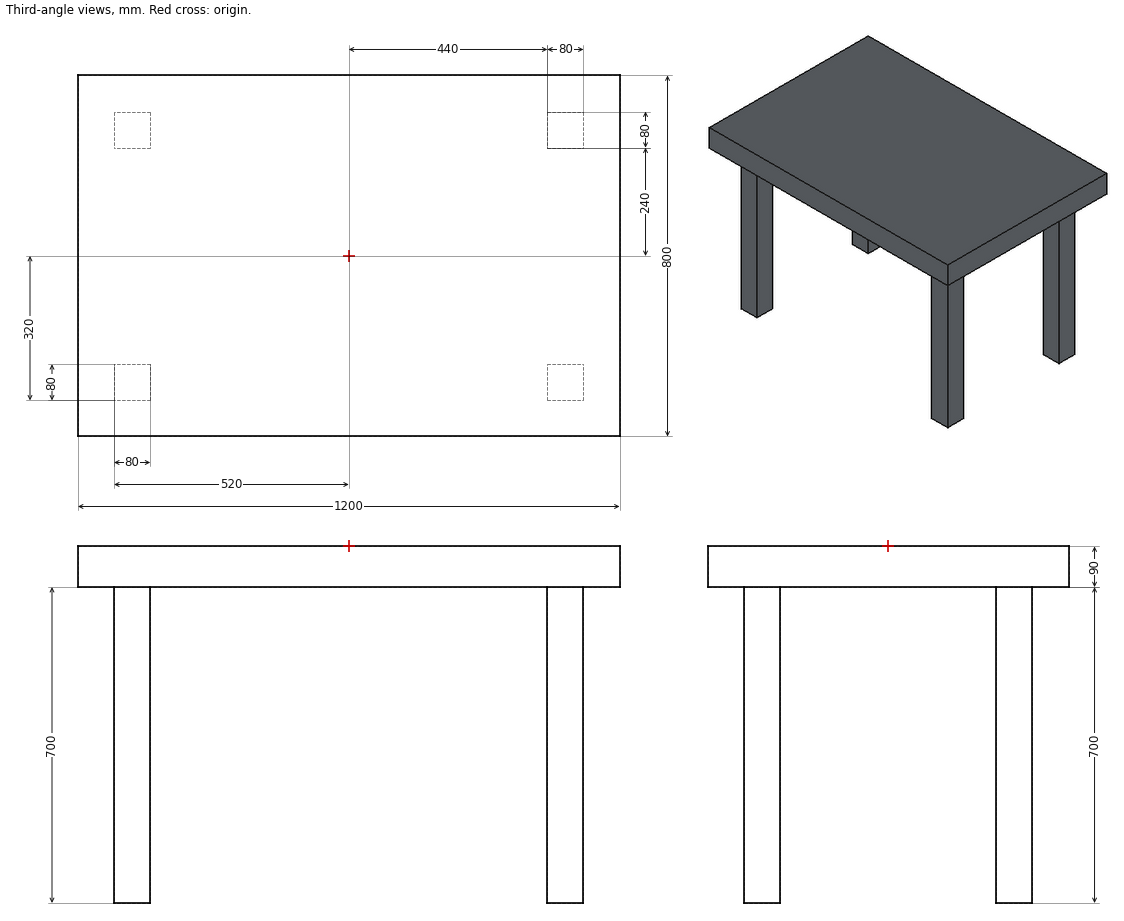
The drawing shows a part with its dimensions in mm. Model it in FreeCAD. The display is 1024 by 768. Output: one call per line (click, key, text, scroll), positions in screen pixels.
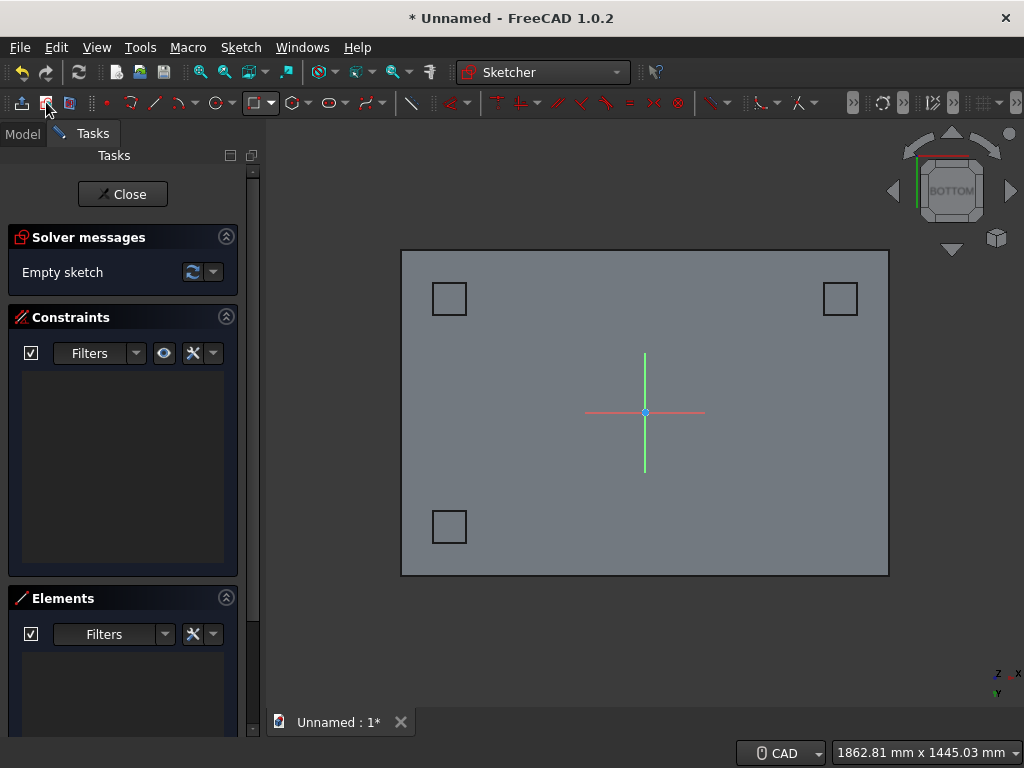
scroll(859, 538, up, 12)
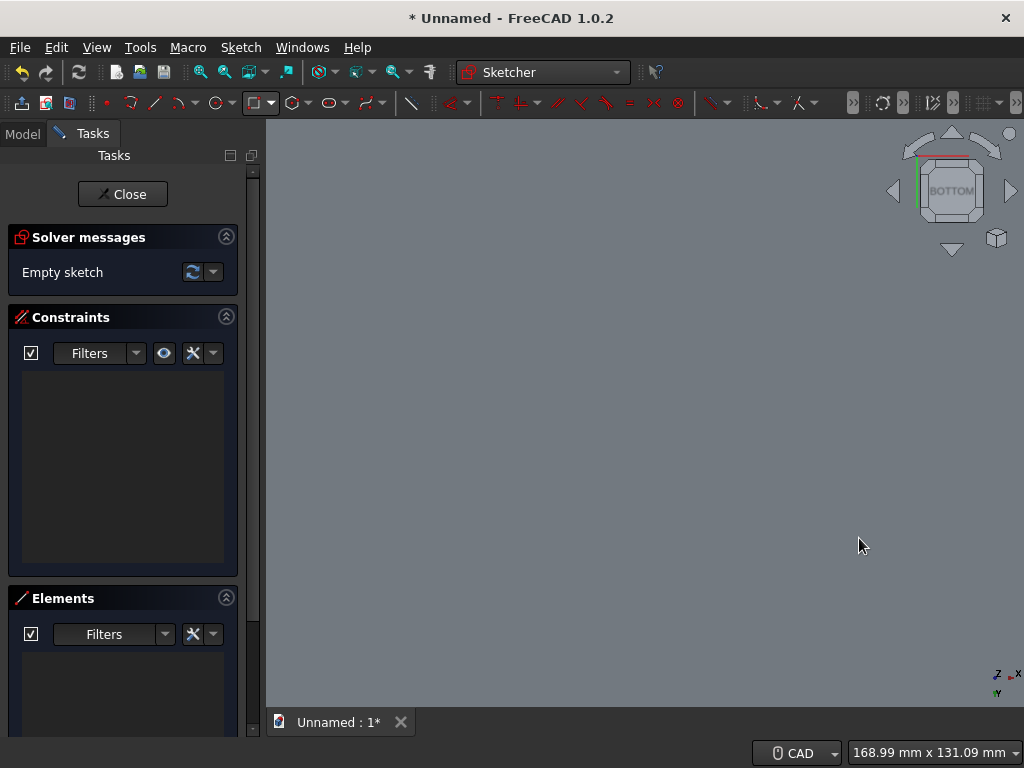
key(g)
key(r)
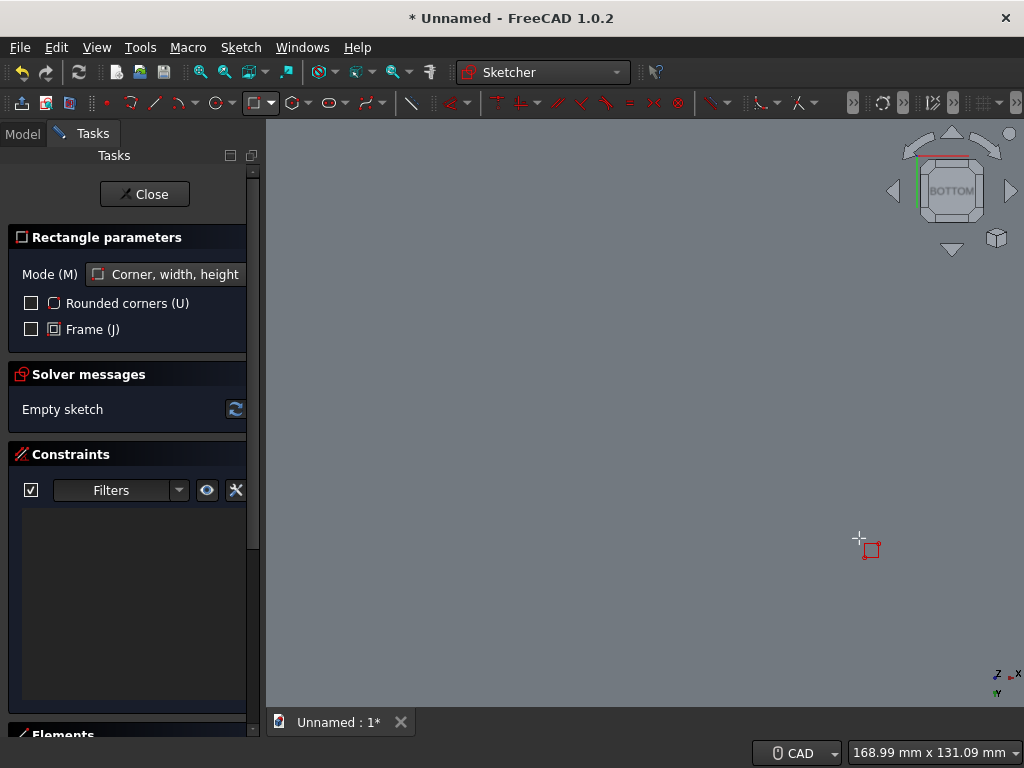
click(466, 229)
click(825, 588)
key(Escape)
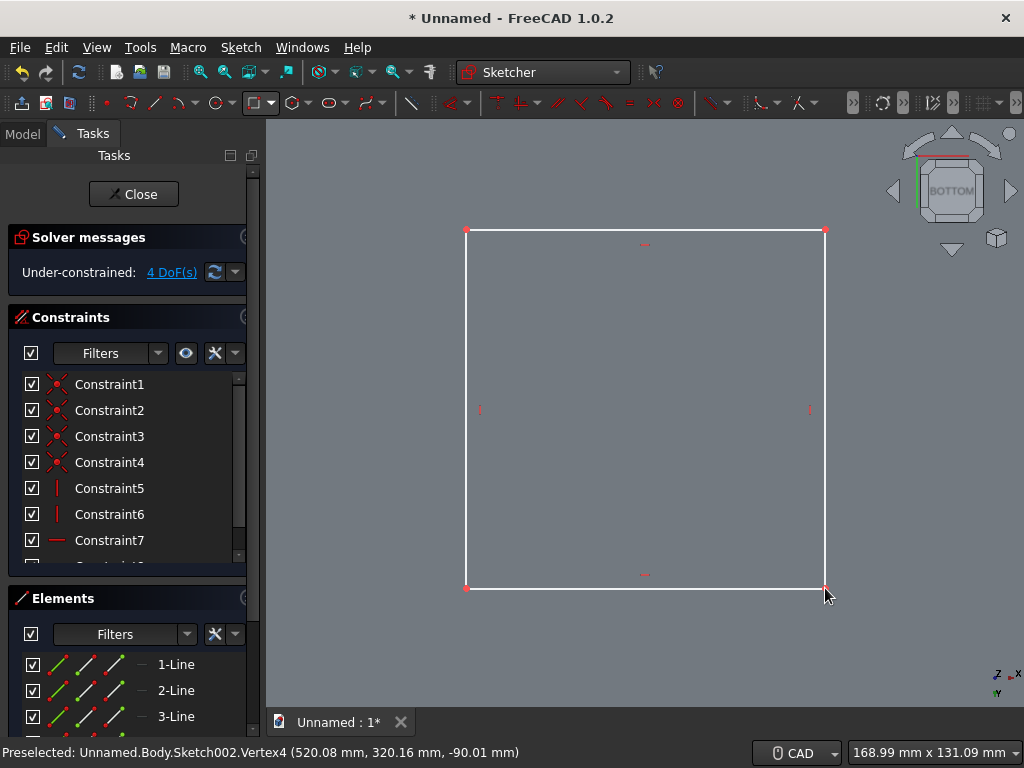
key(d)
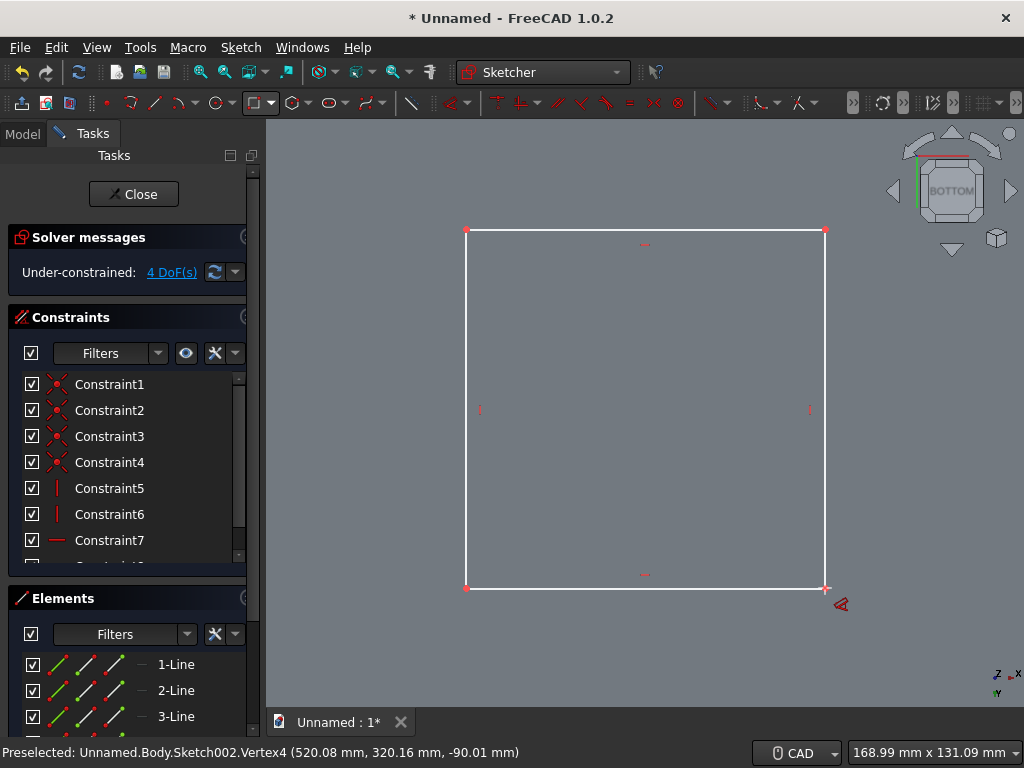
click(466, 338)
click(432, 410)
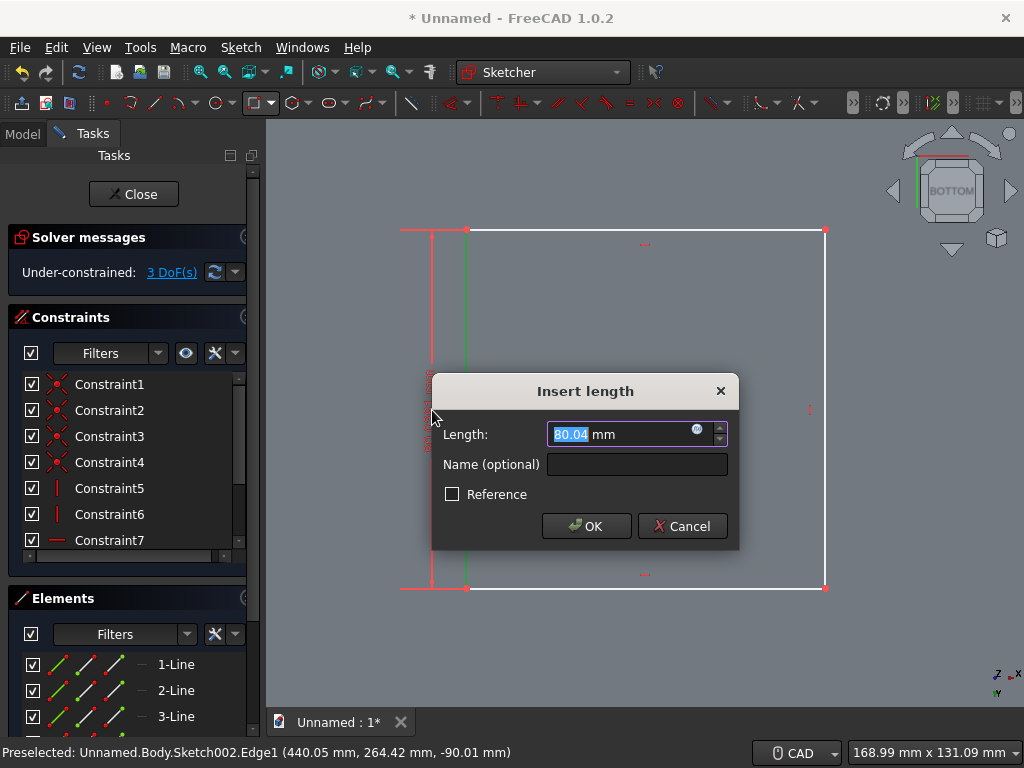
text(80)
key(Return)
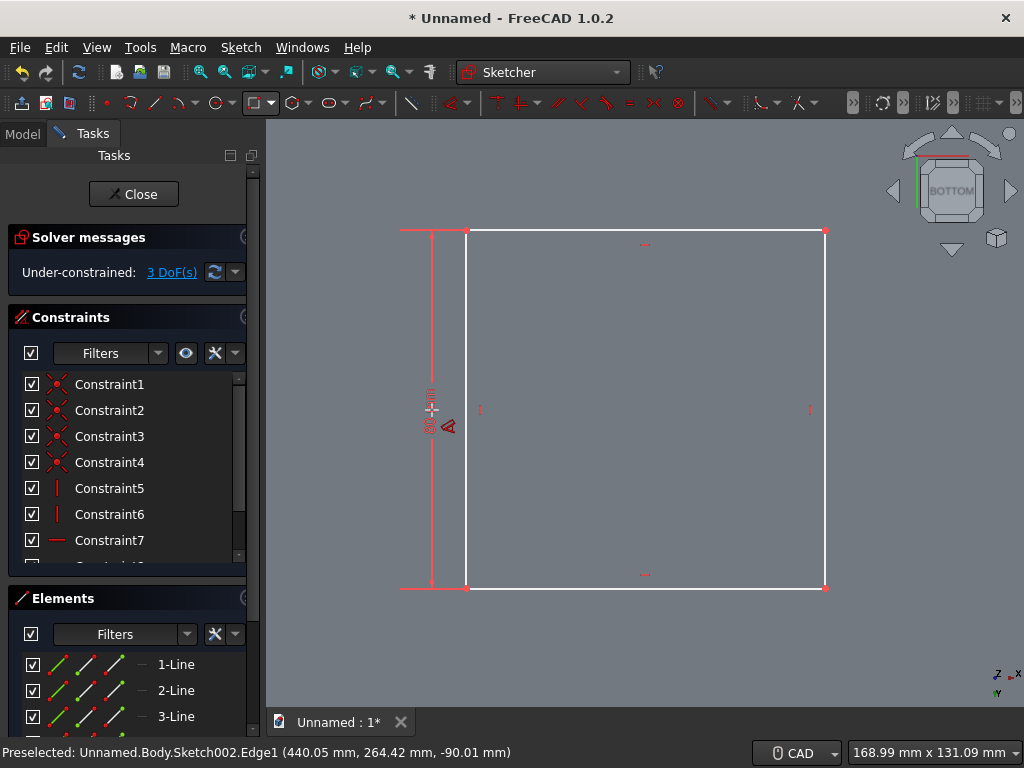
click(574, 589)
click(645, 623)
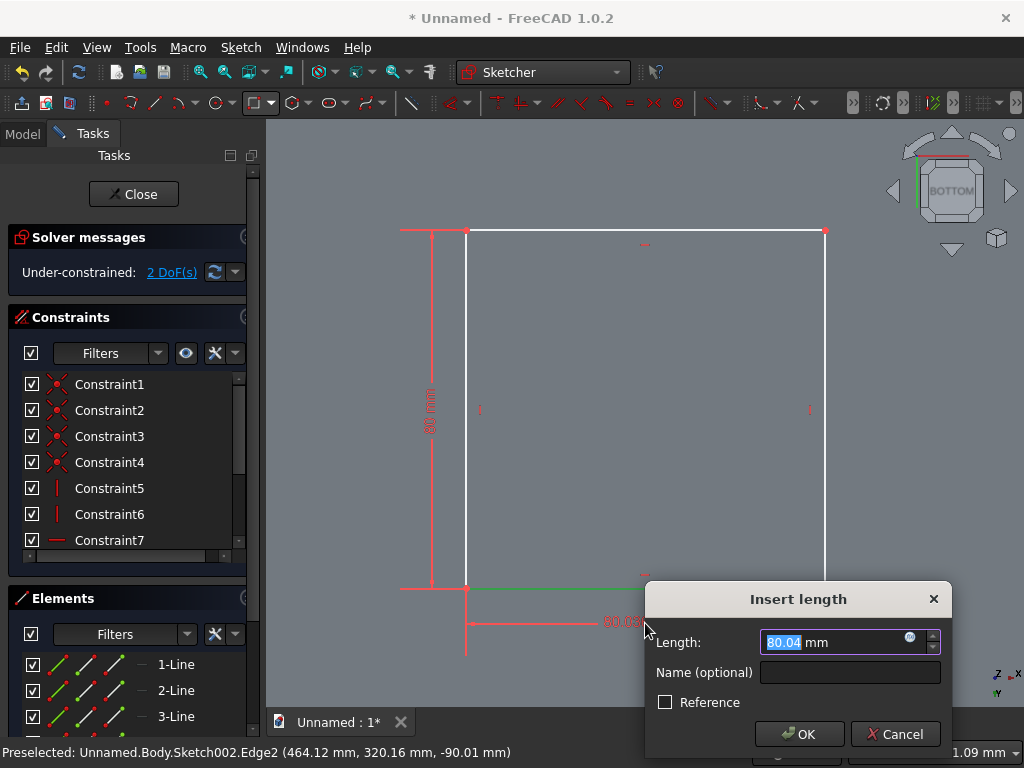
text(80)
key(Return)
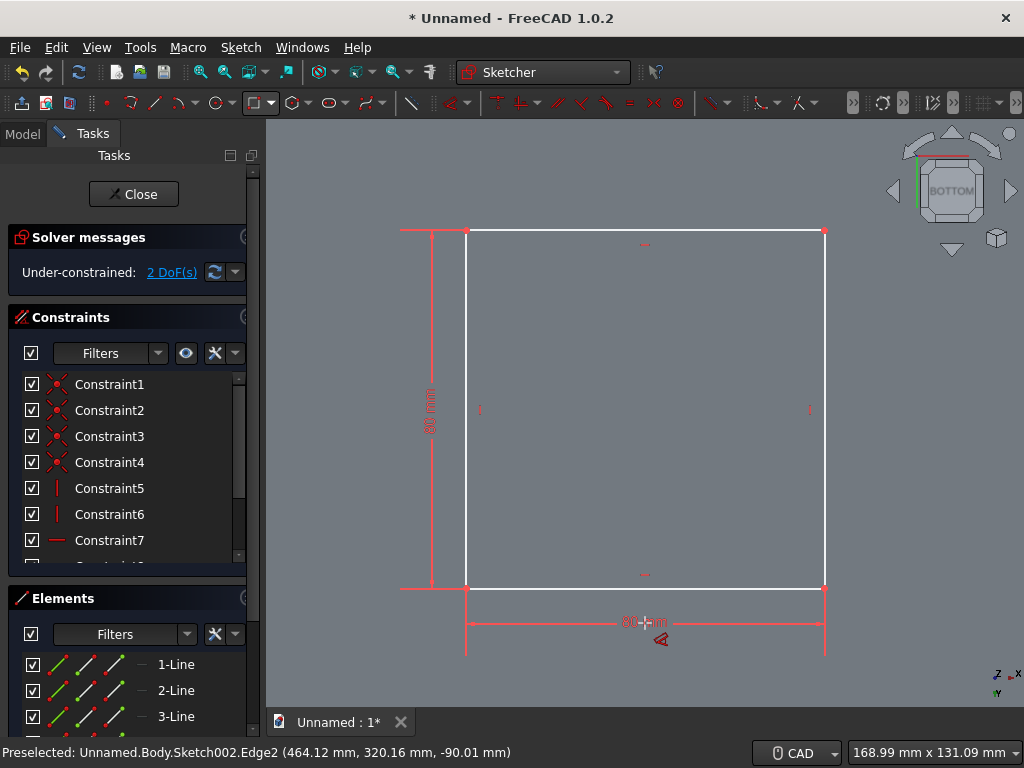
click(466, 230)
click(380, 264)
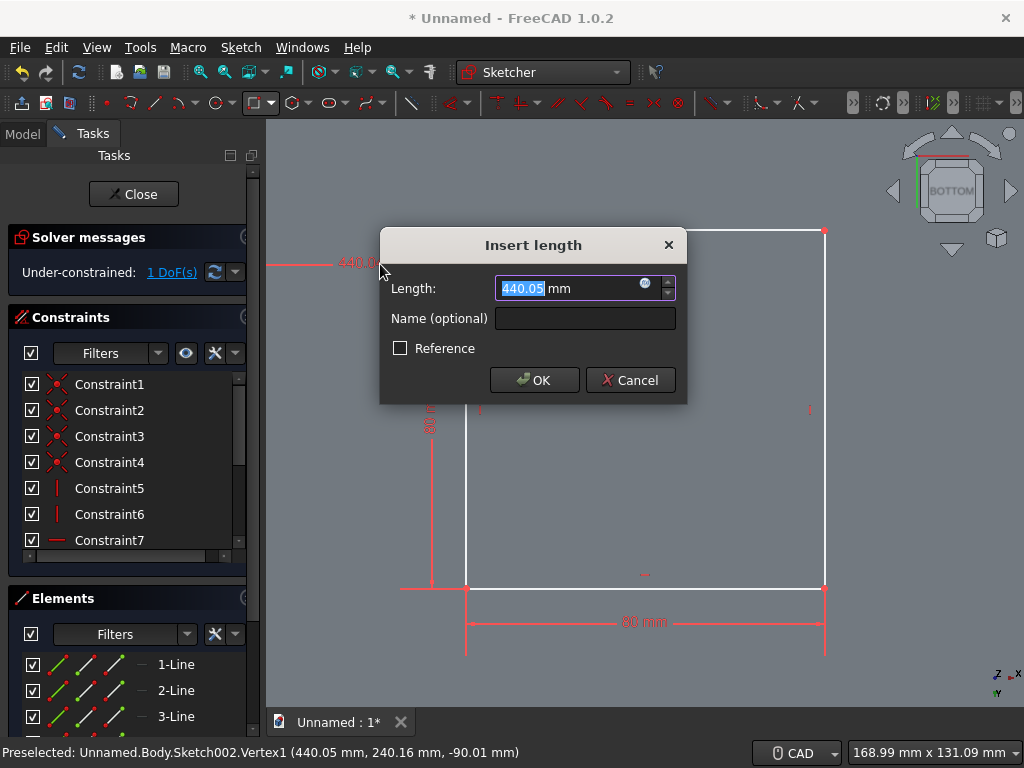
text(440)
key(Return)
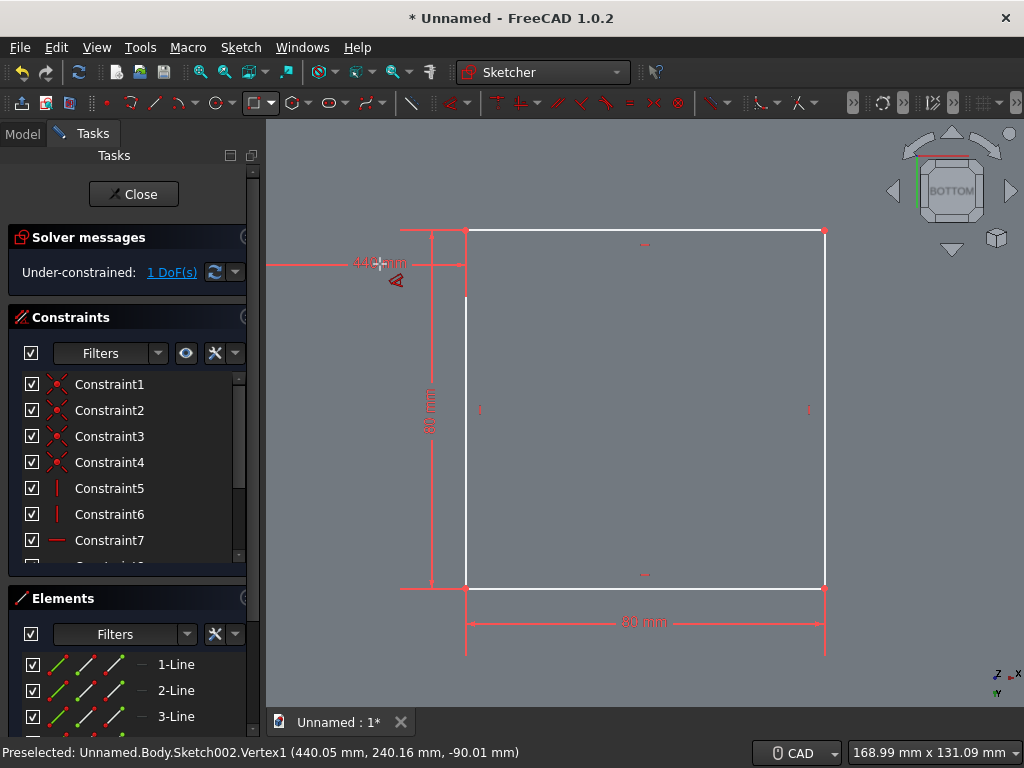
click(466, 230)
click(500, 189)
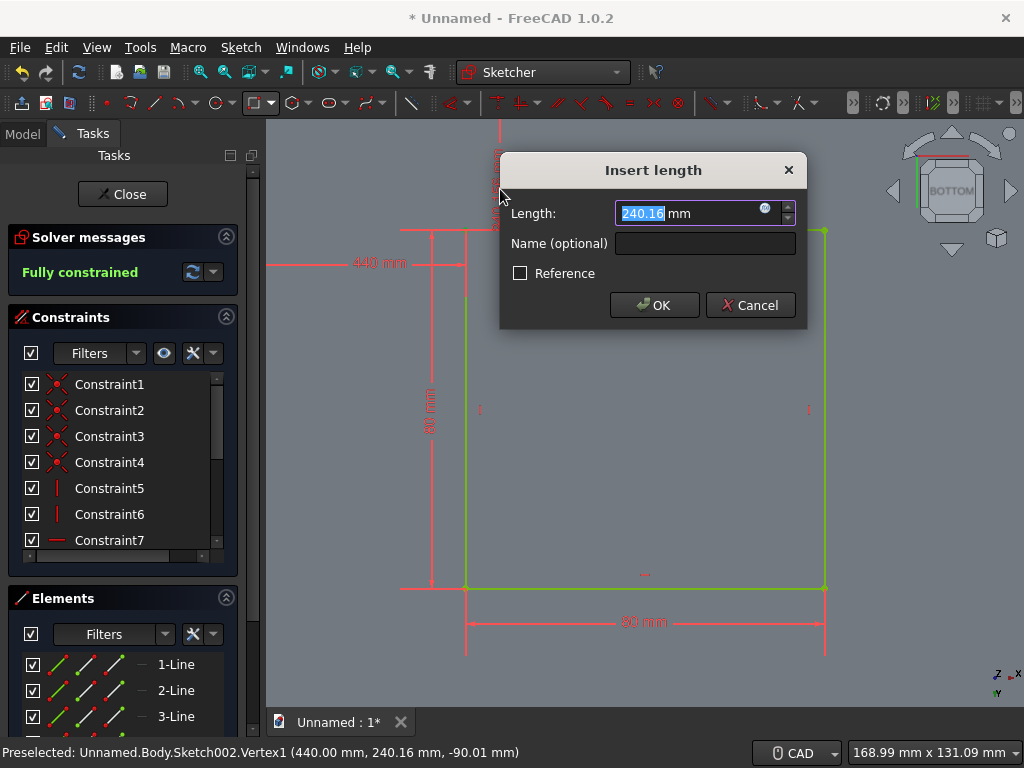
text(240)
key(Return)
key(Escape)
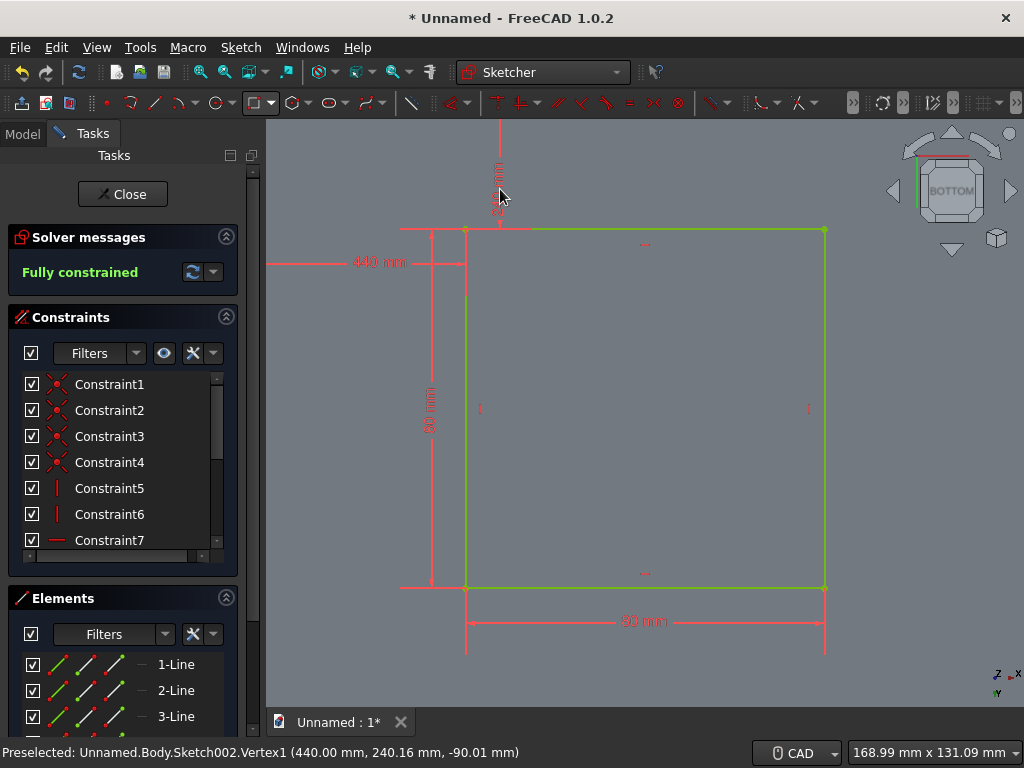
click(123, 194)